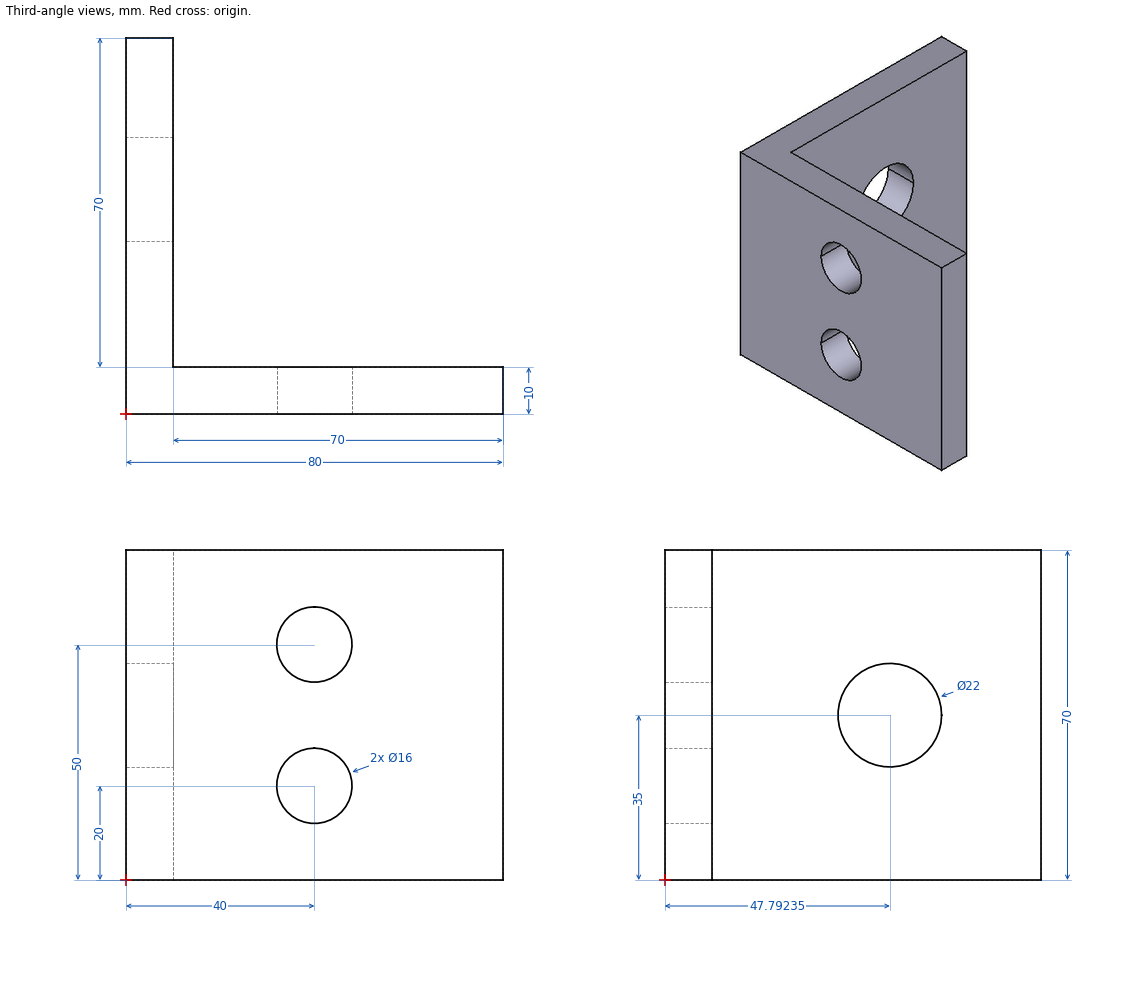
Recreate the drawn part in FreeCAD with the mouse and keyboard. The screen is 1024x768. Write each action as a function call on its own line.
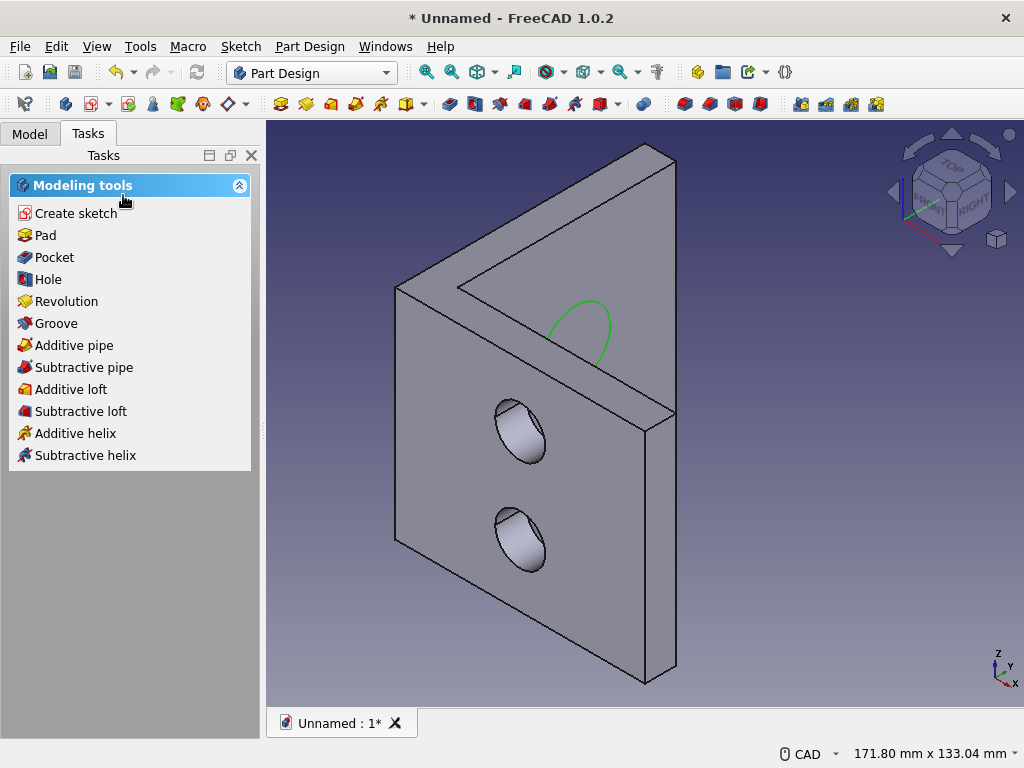
click(450, 104)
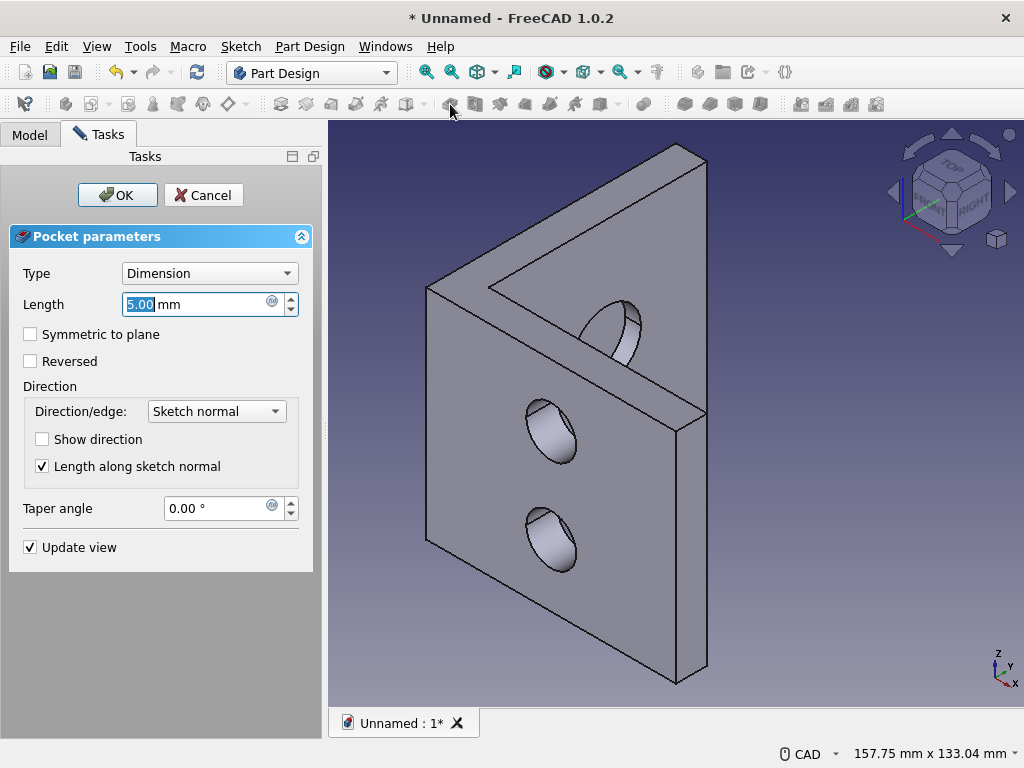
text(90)
key(Tab)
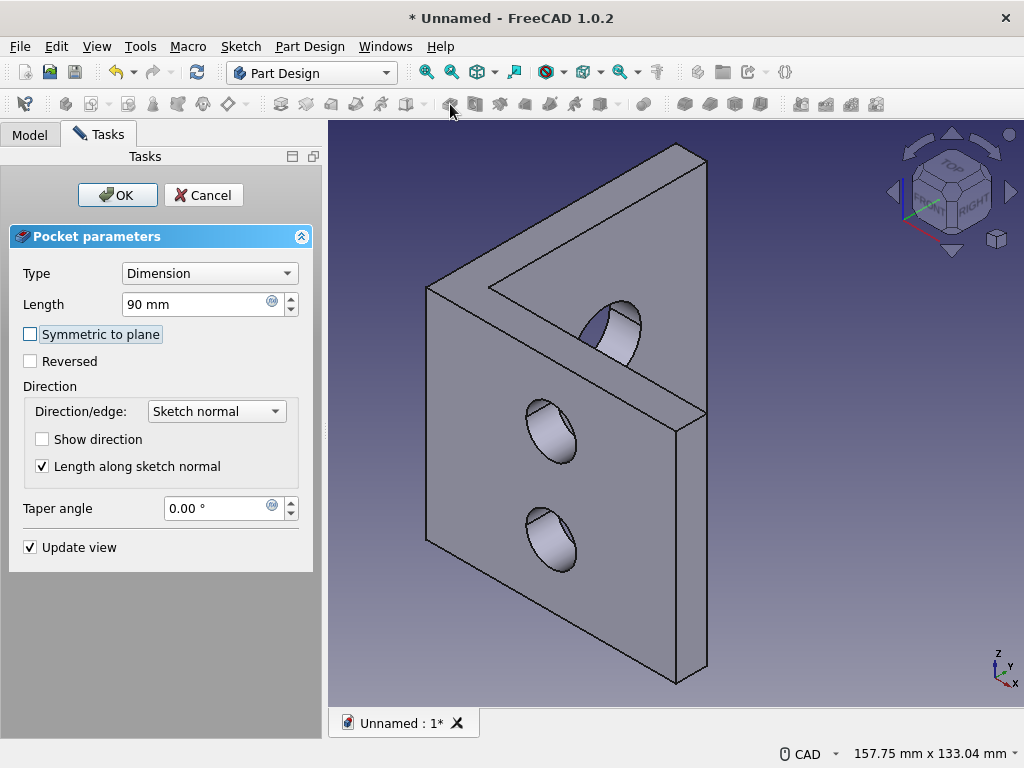
click(118, 195)